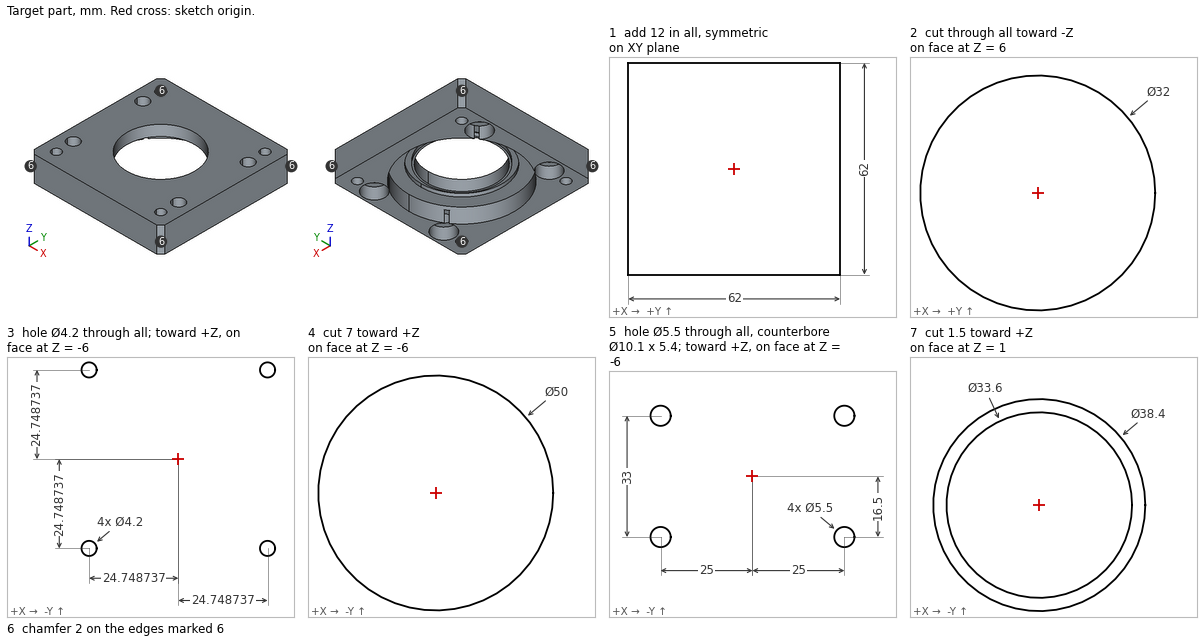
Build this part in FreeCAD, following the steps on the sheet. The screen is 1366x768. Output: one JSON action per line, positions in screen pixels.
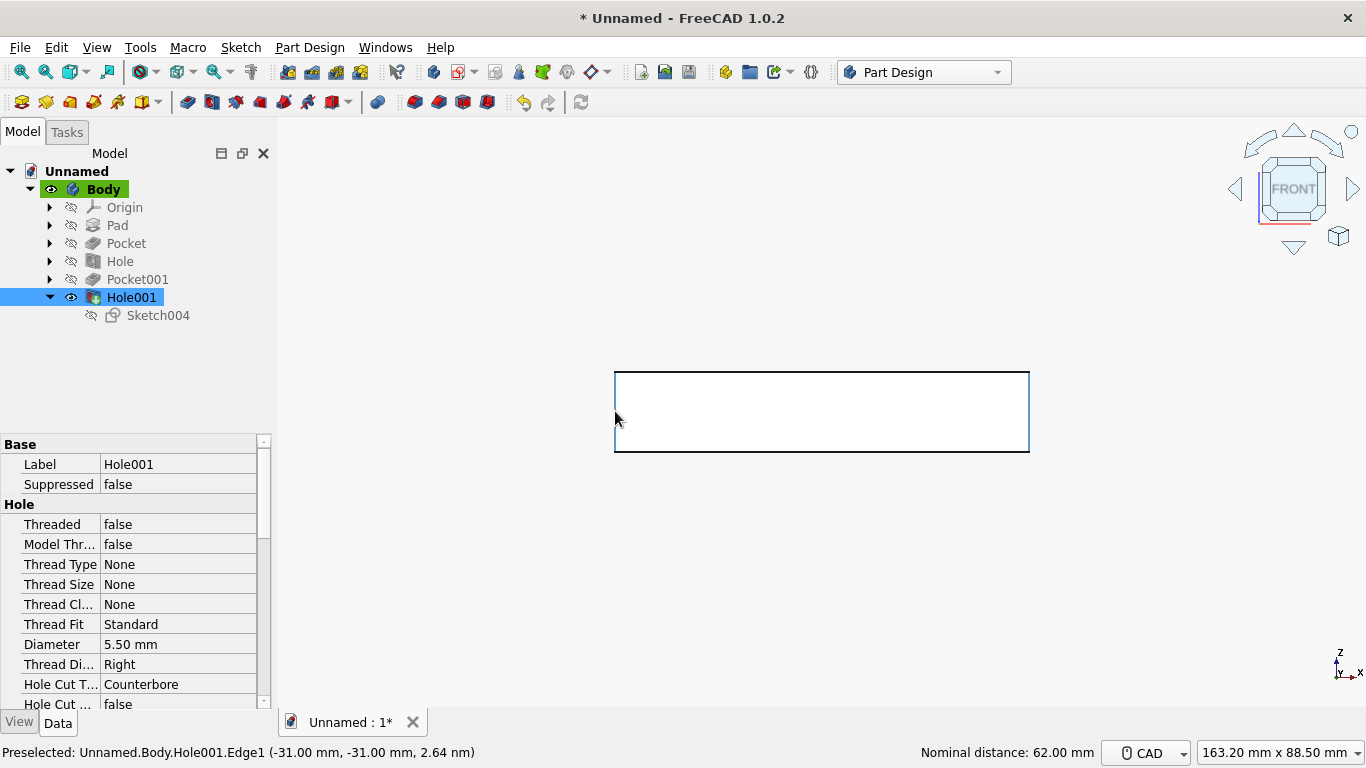
{"action": "key", "text": "3"}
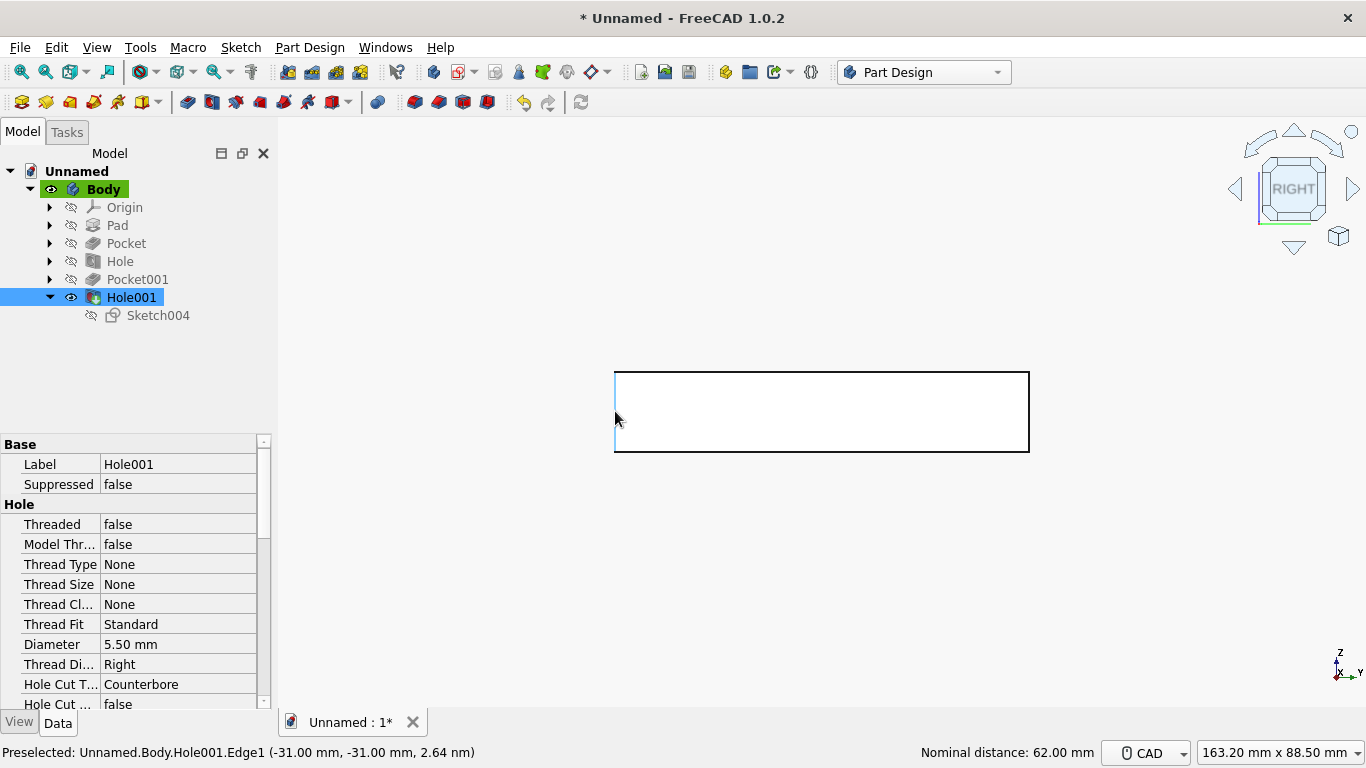
{"action": "left_click", "coordinate": [22, 72]}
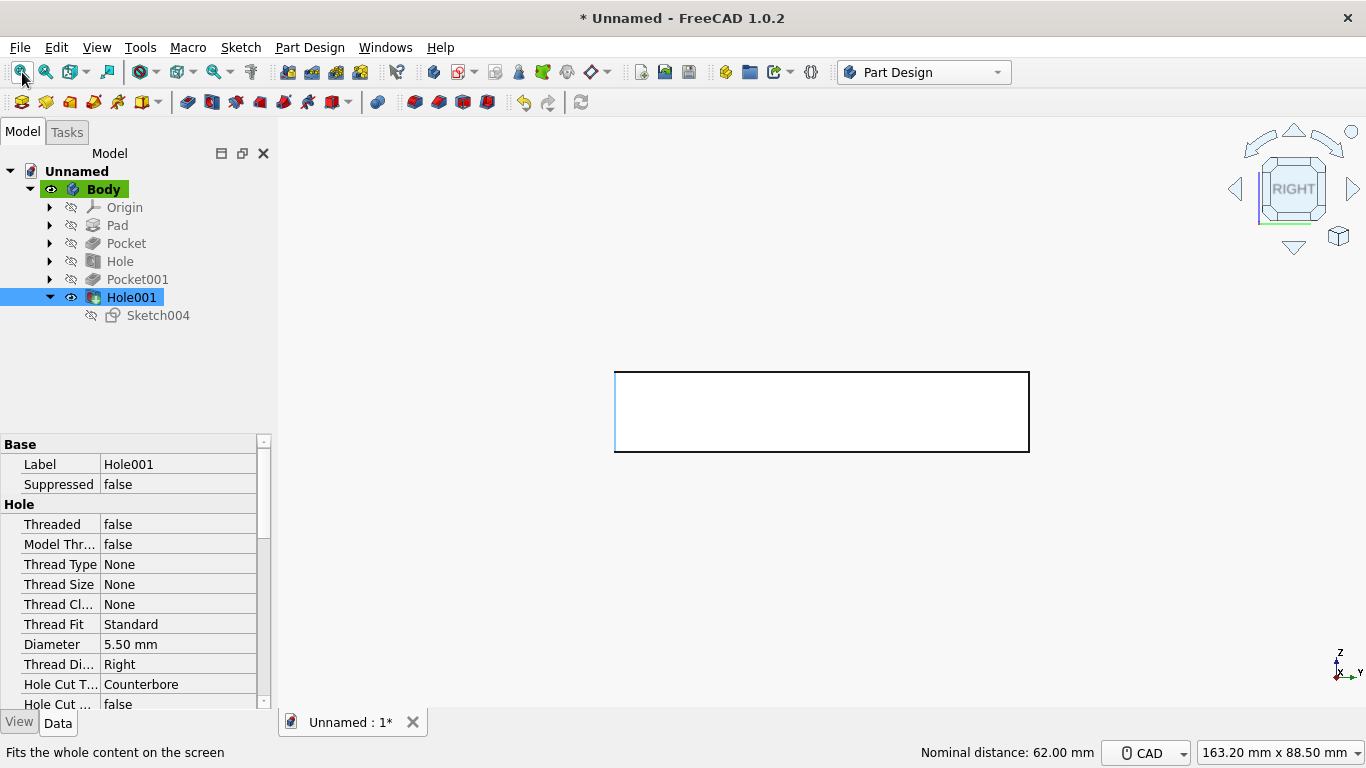
{"action": "left_click", "coordinate": [1029, 411], "text": "ctrl"}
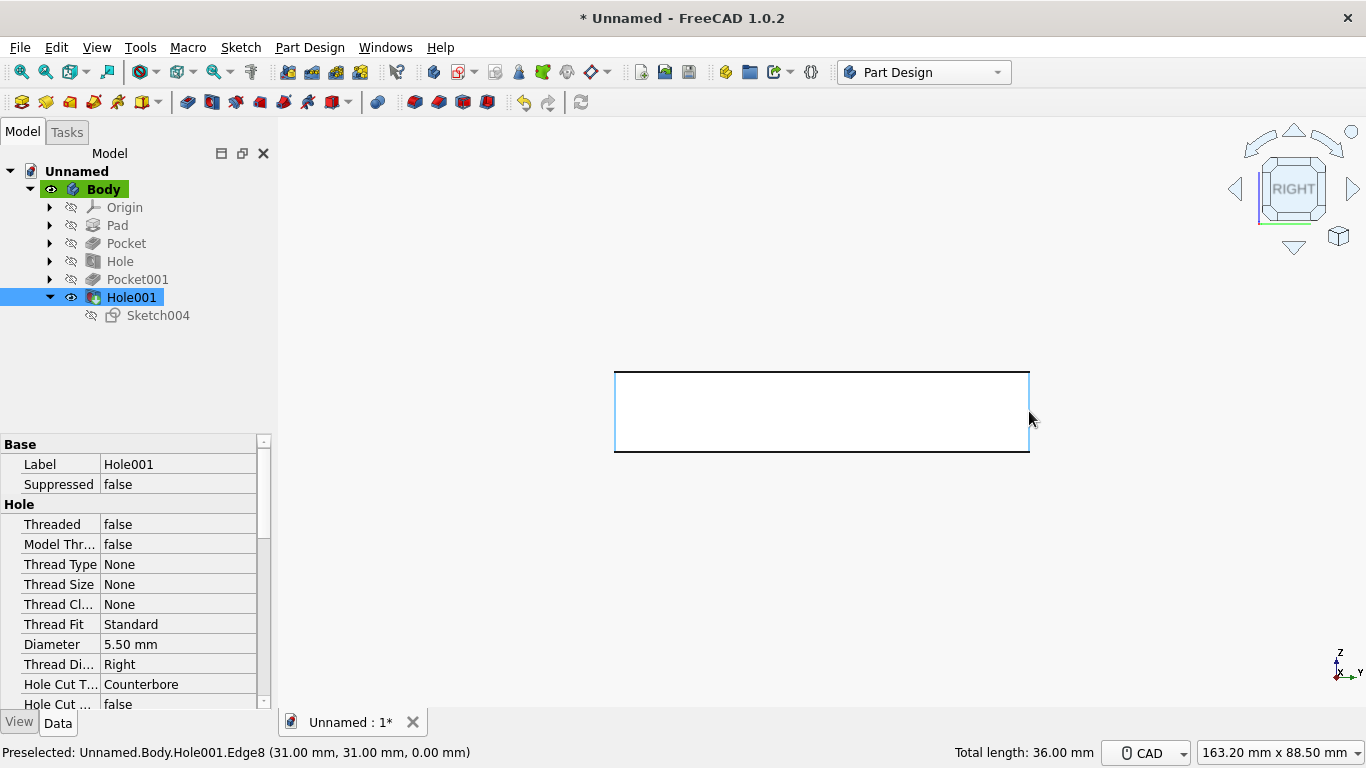
{"action": "key", "text": "5"}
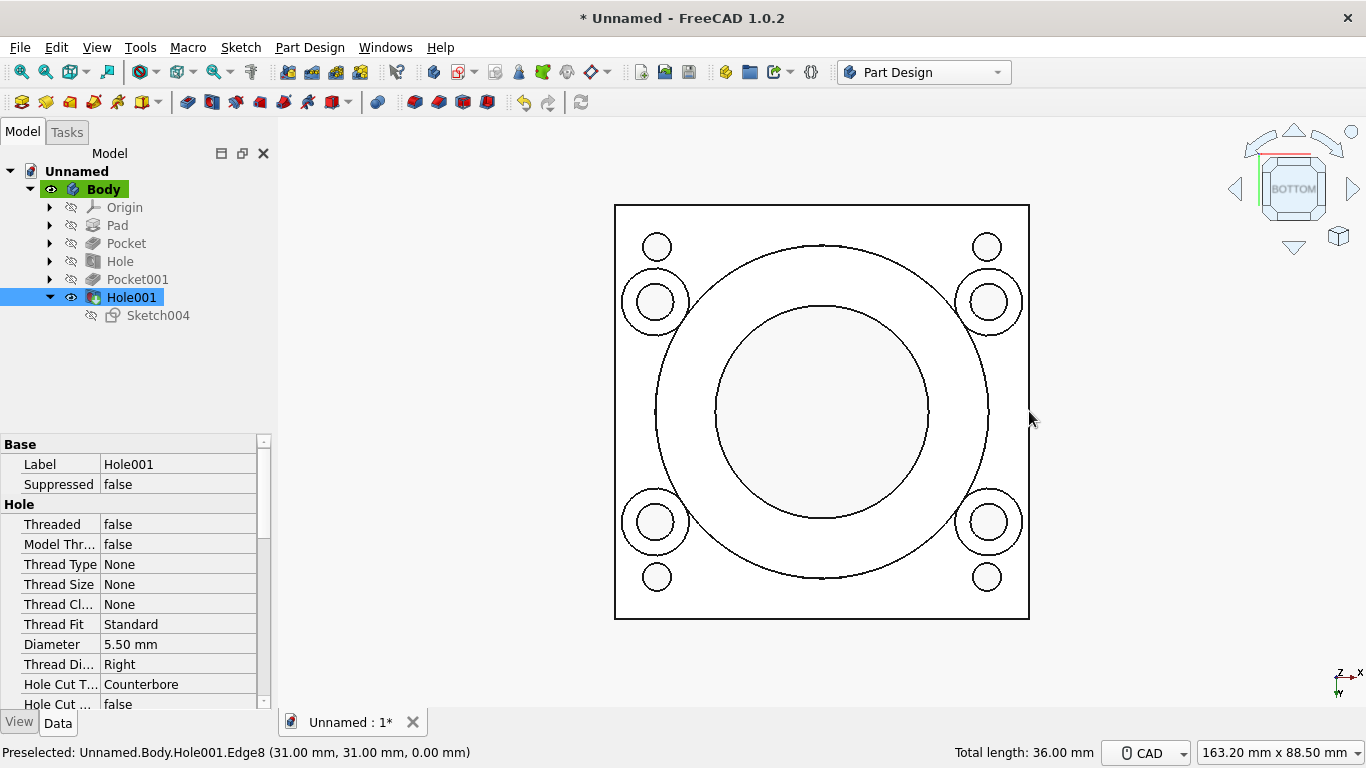
{"action": "key", "text": "4"}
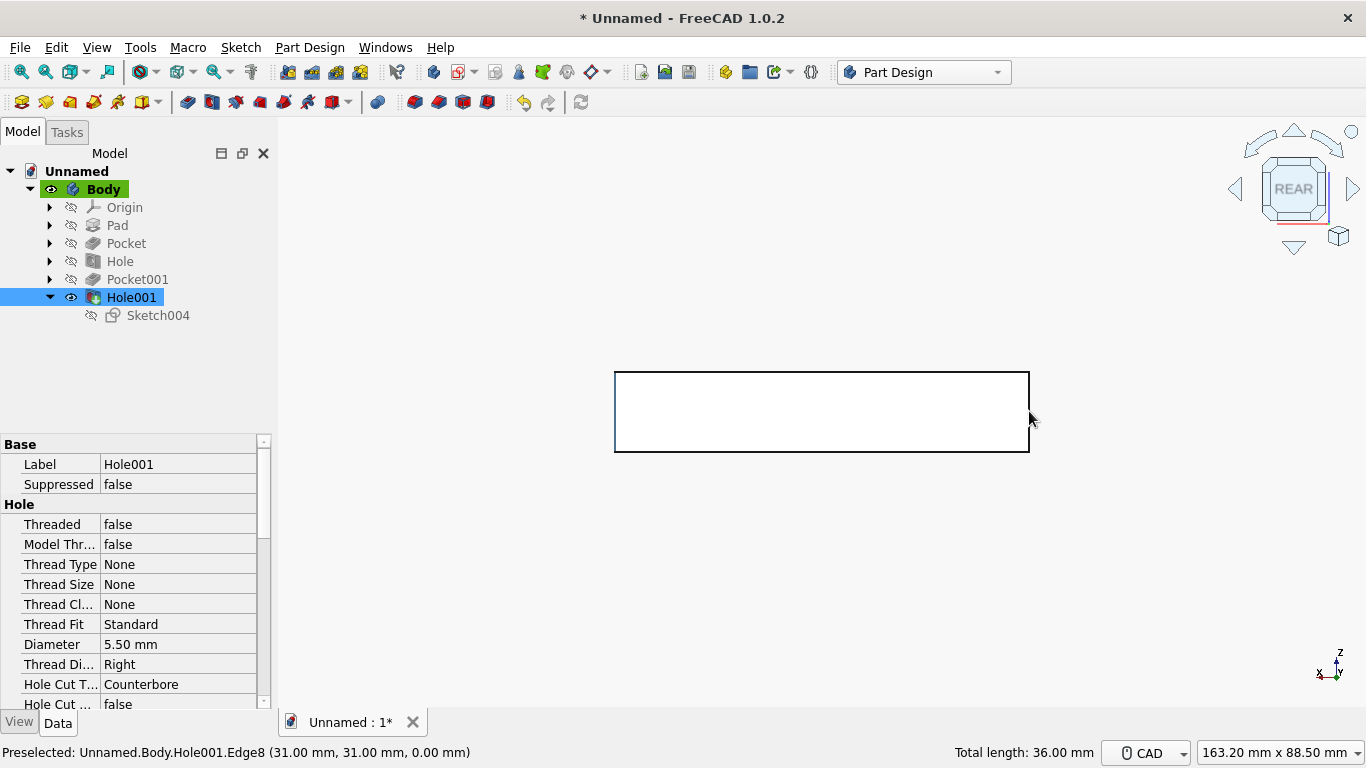
{"action": "left_click", "coordinate": [22, 72]}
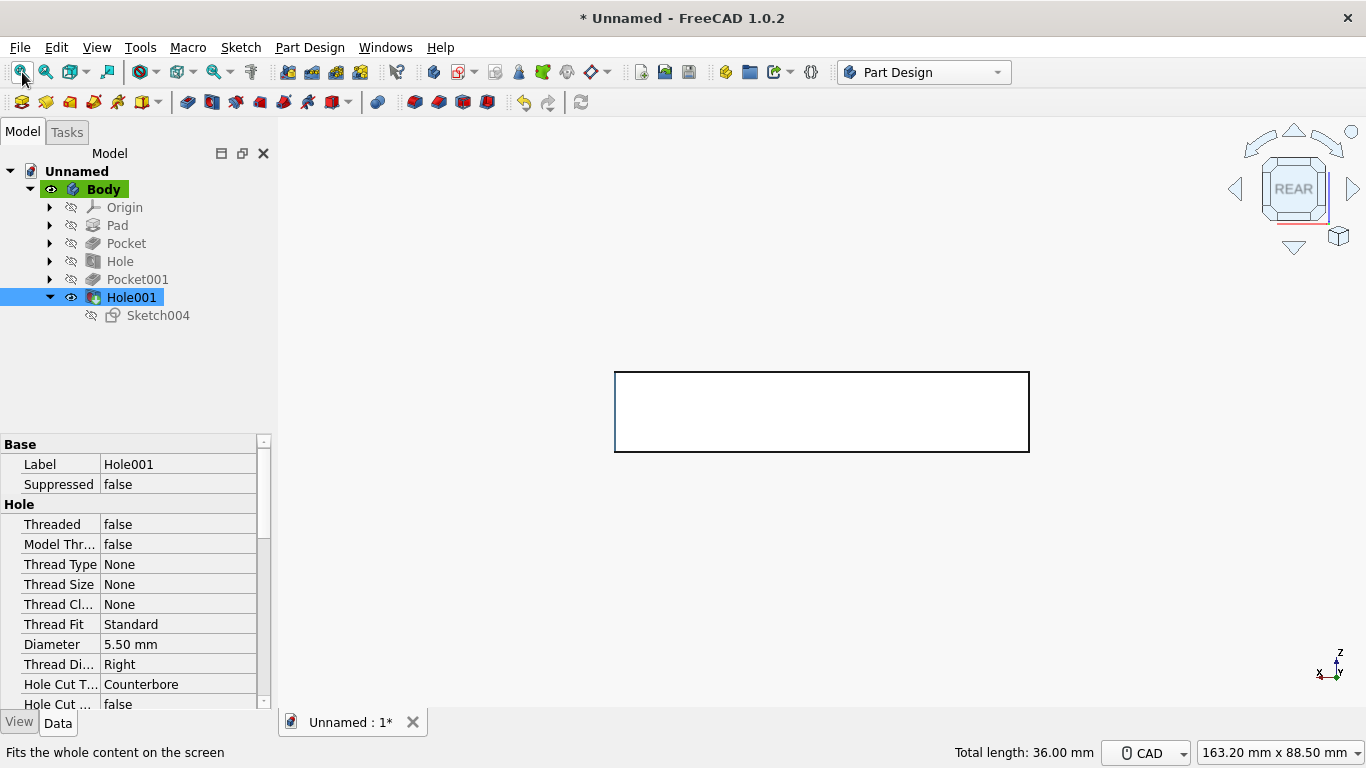
{"action": "left_click", "coordinate": [1029, 411], "text": "ctrl"}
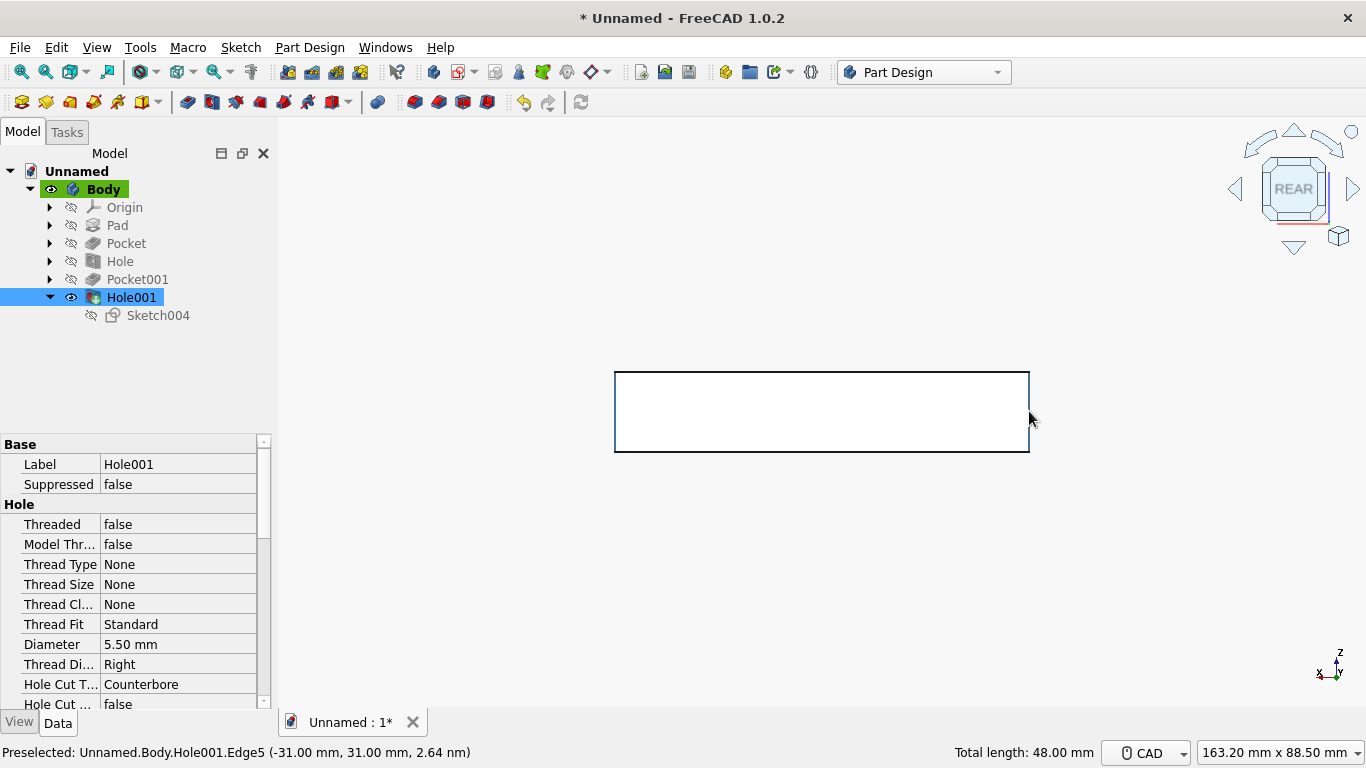
{"action": "left_click", "coordinate": [440, 102]}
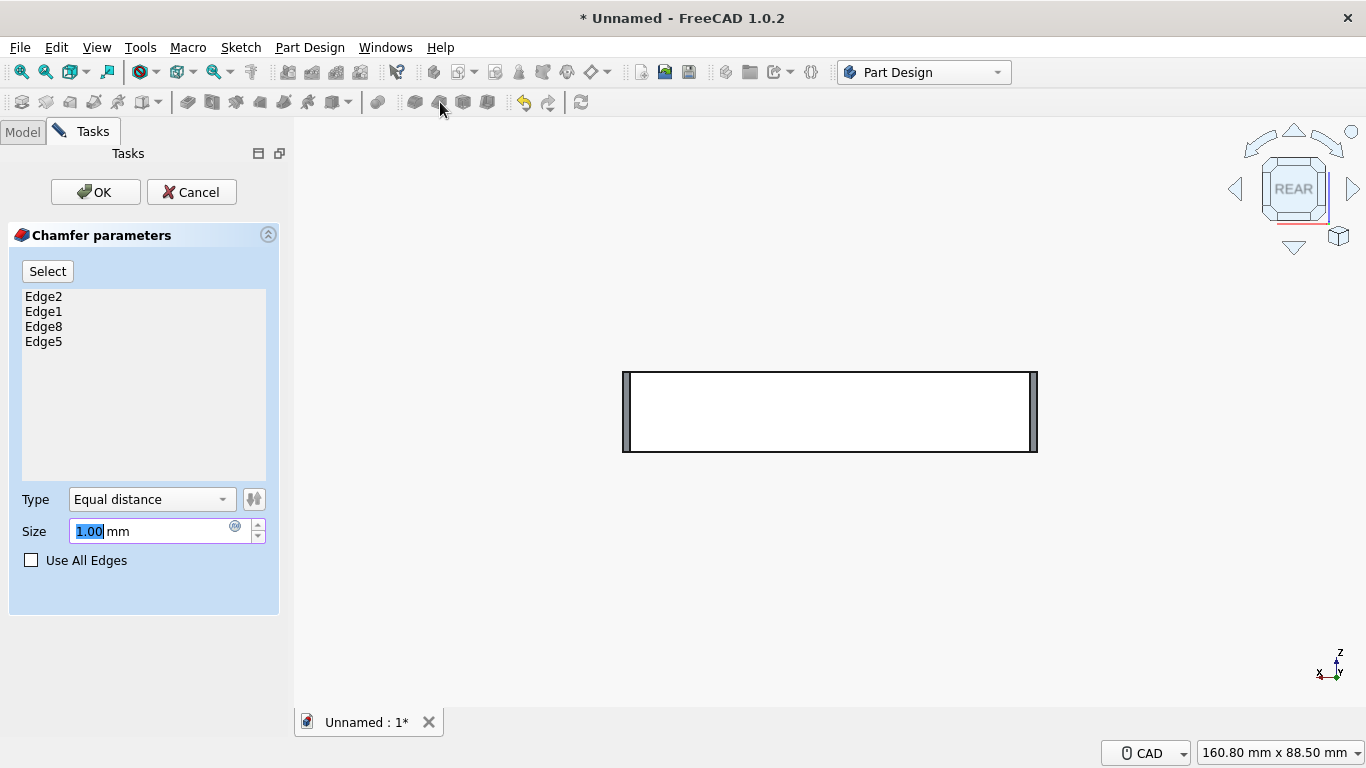
{"action": "type", "text": "2"}
{"action": "key", "text": "Tab"}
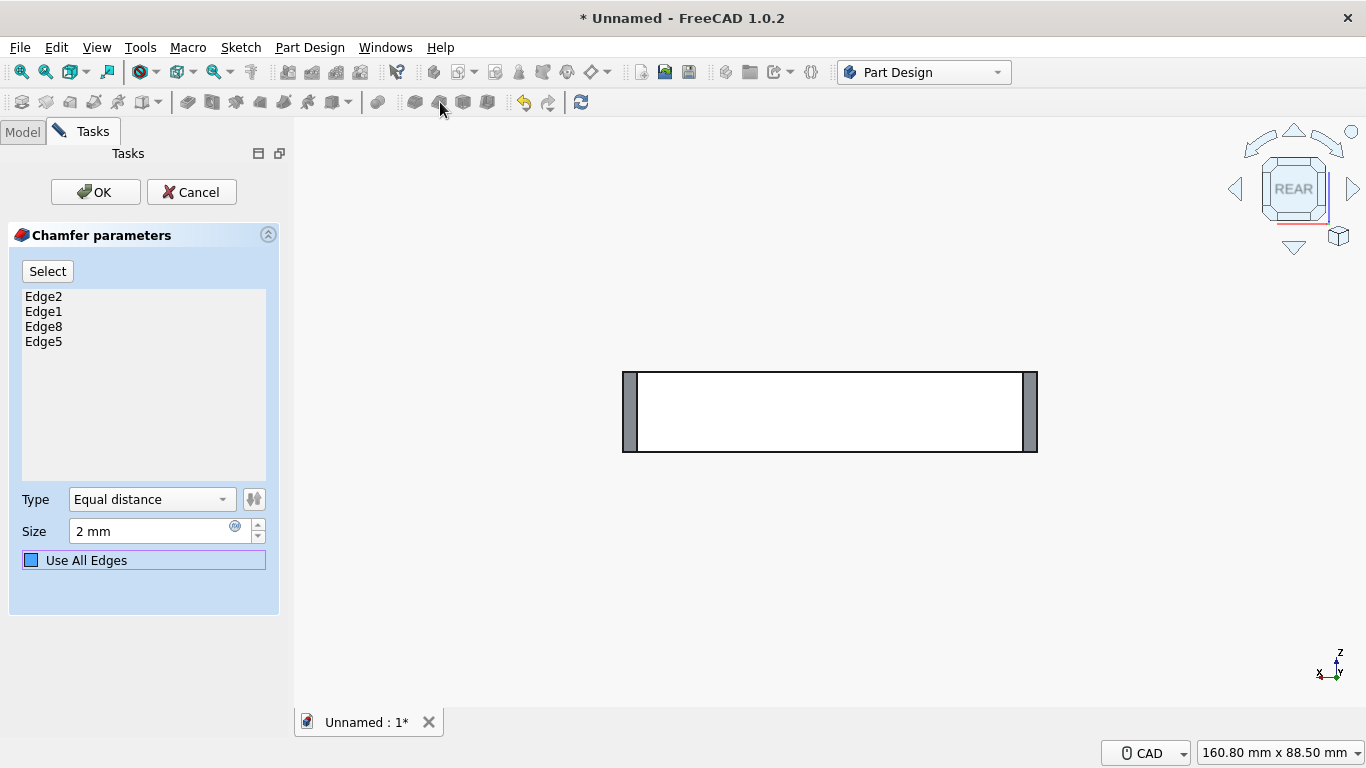
{"action": "left_click", "coordinate": [96, 192]}